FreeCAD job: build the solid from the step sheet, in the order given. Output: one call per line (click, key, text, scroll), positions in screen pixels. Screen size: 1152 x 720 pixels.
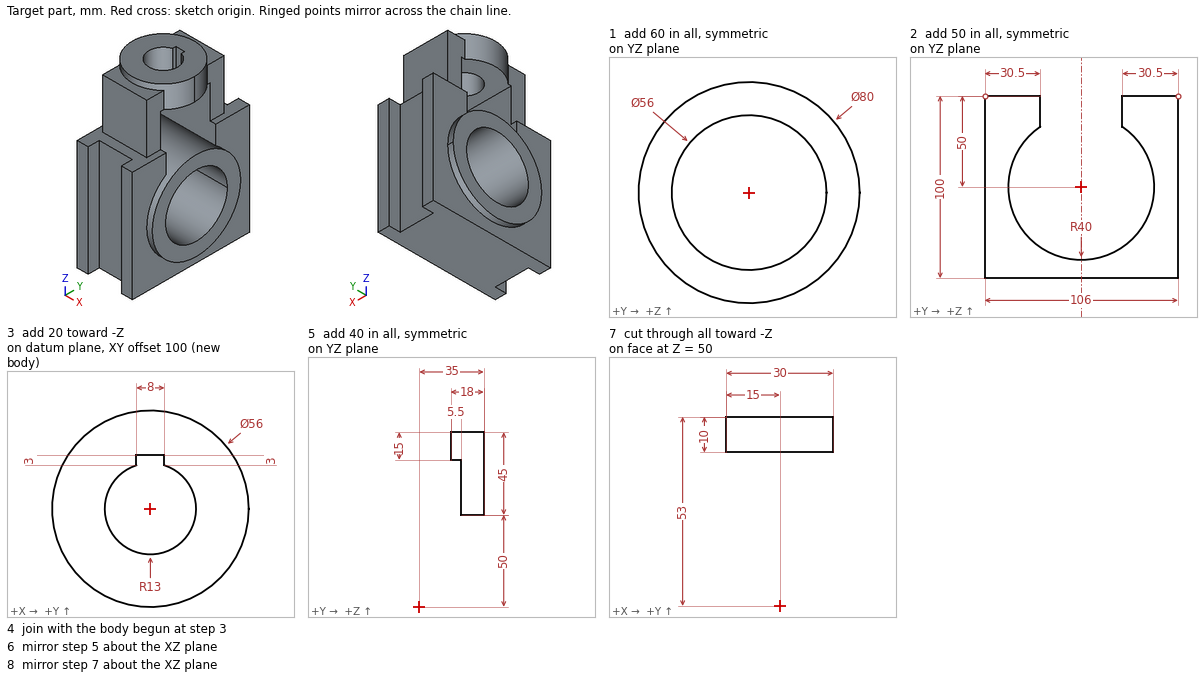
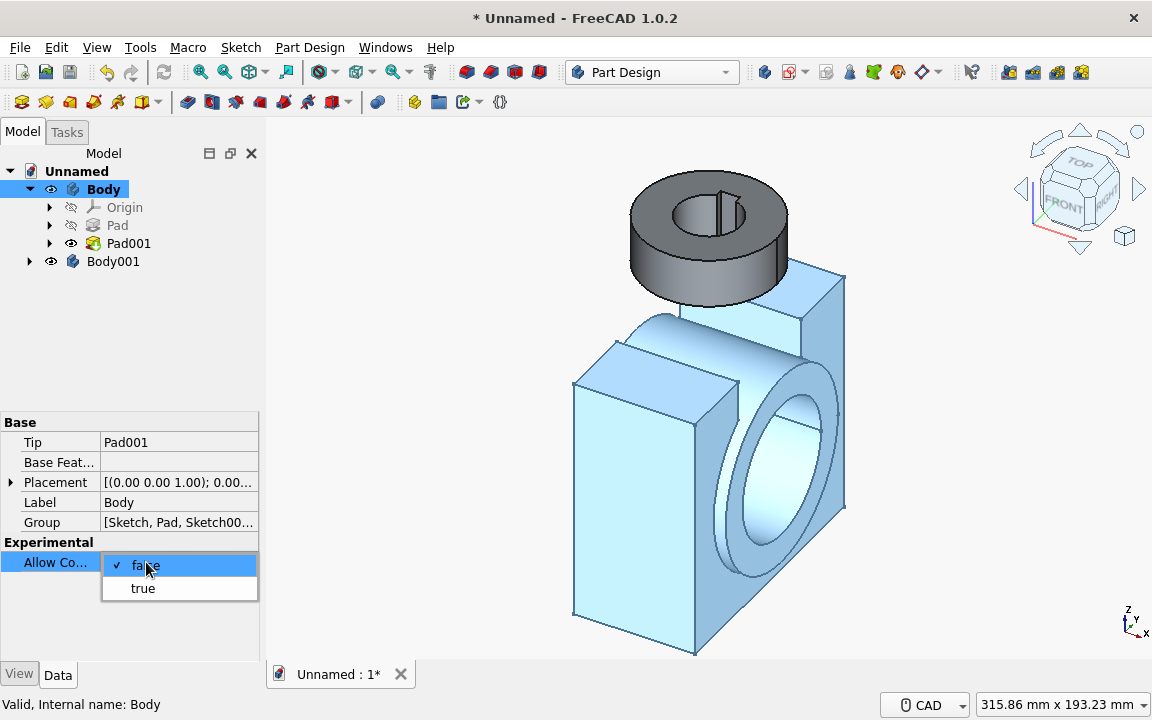
click(179, 588)
key(Return)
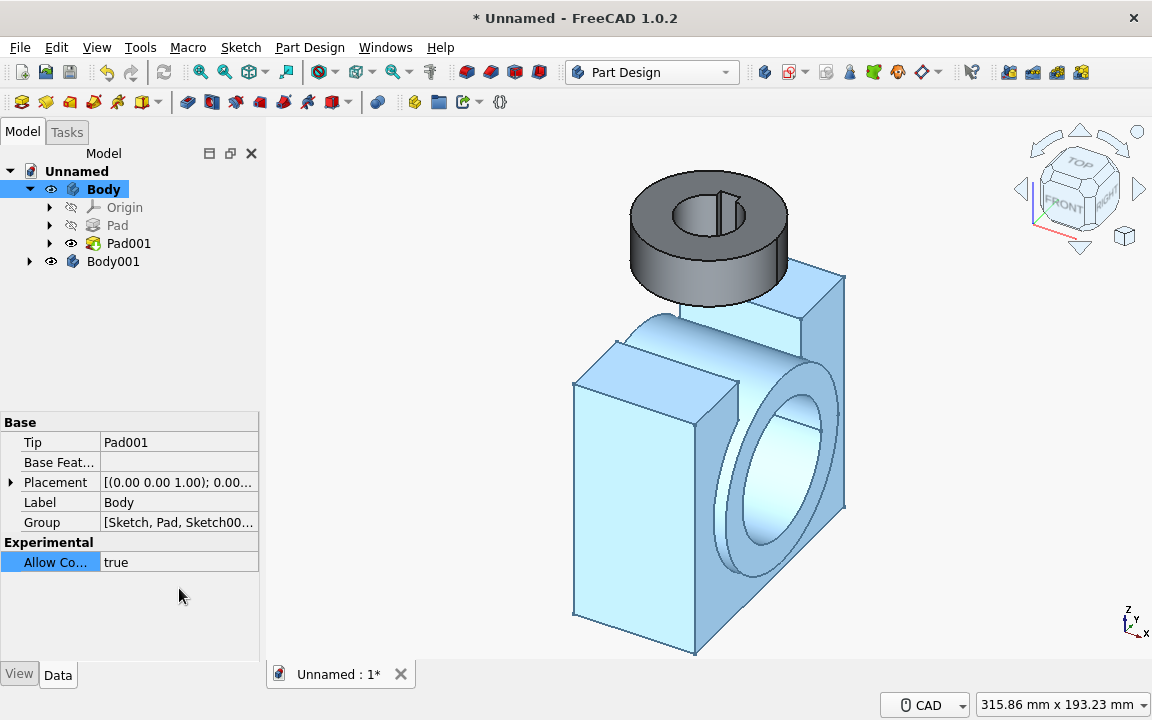
click(96, 261)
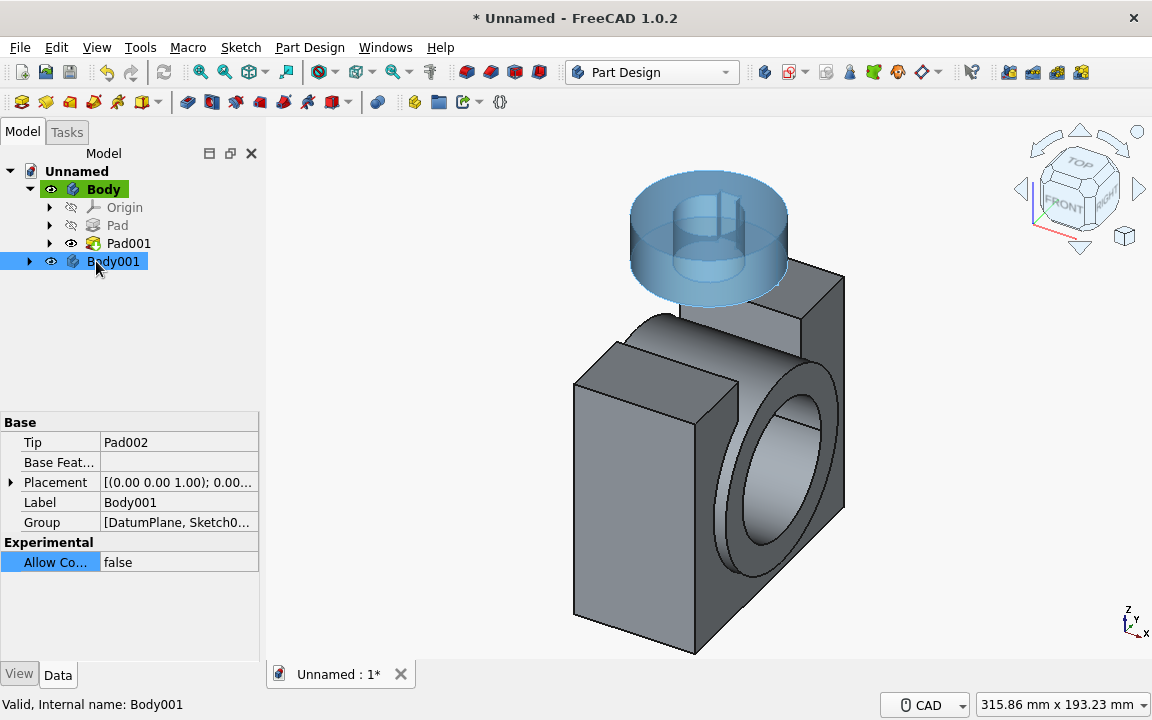
click(378, 102)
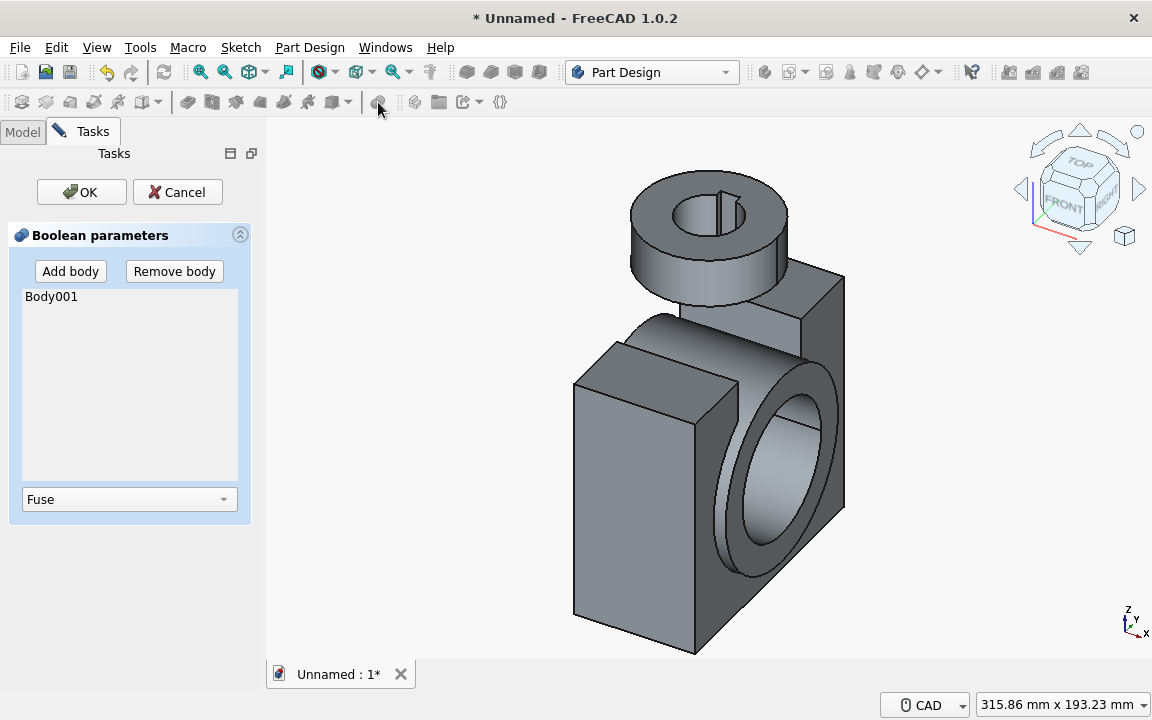
click(82, 192)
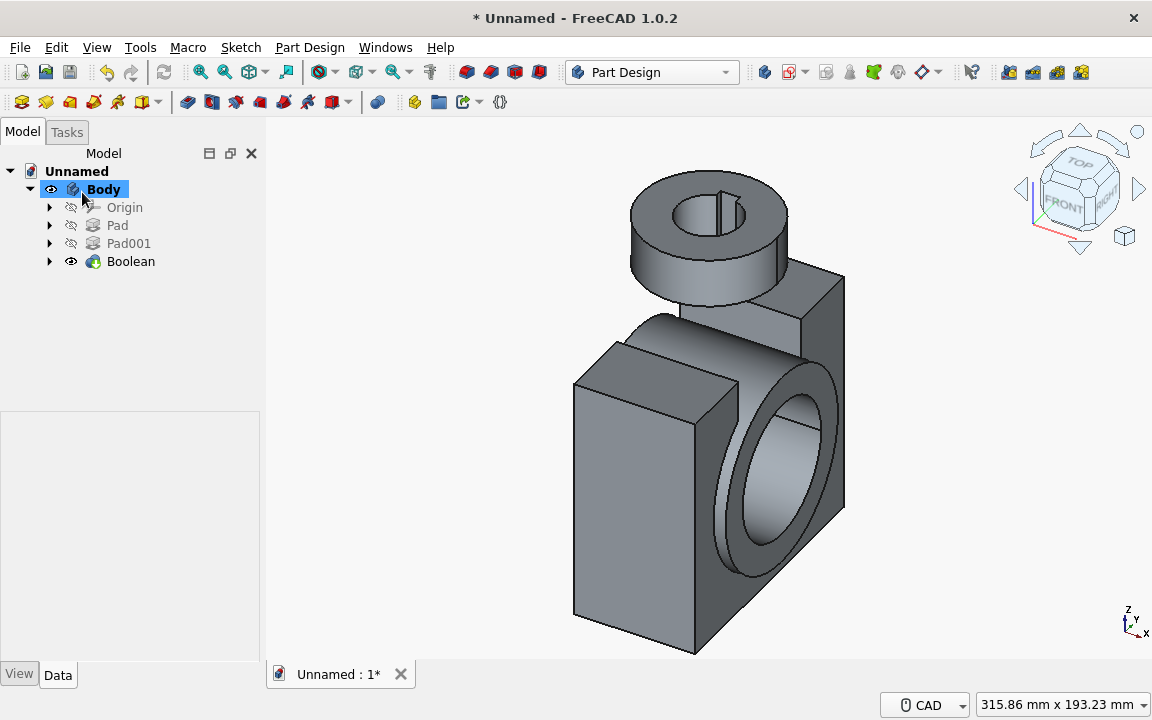
click(790, 72)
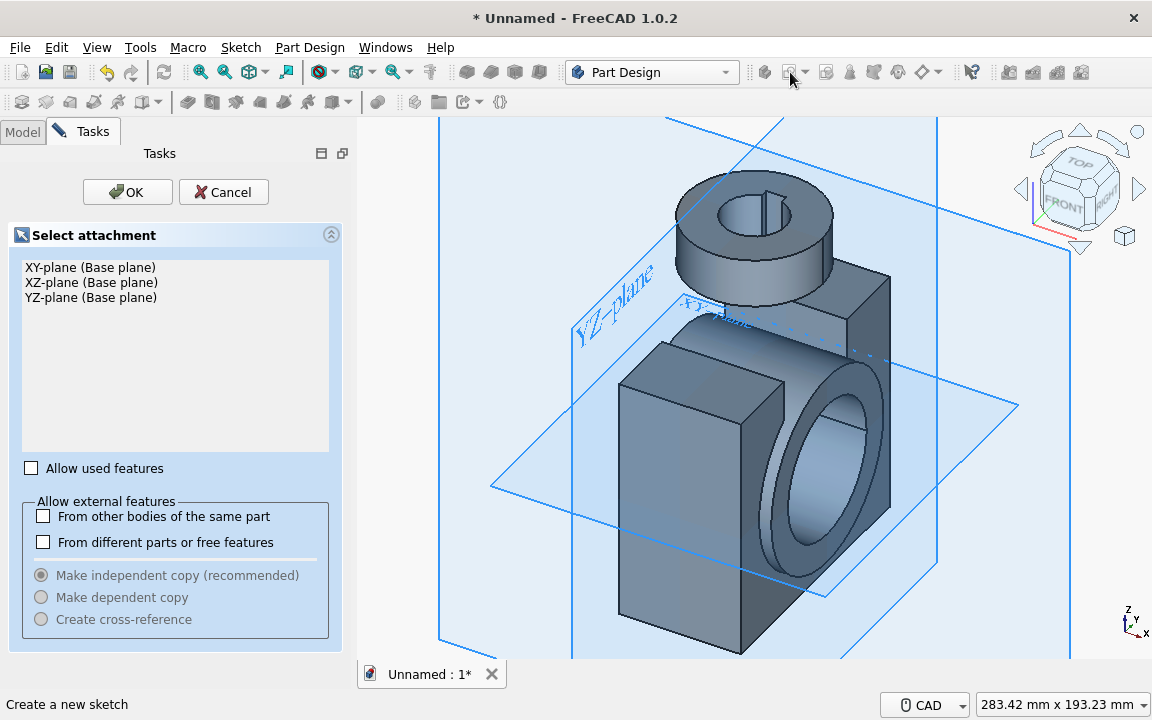
click(82, 298)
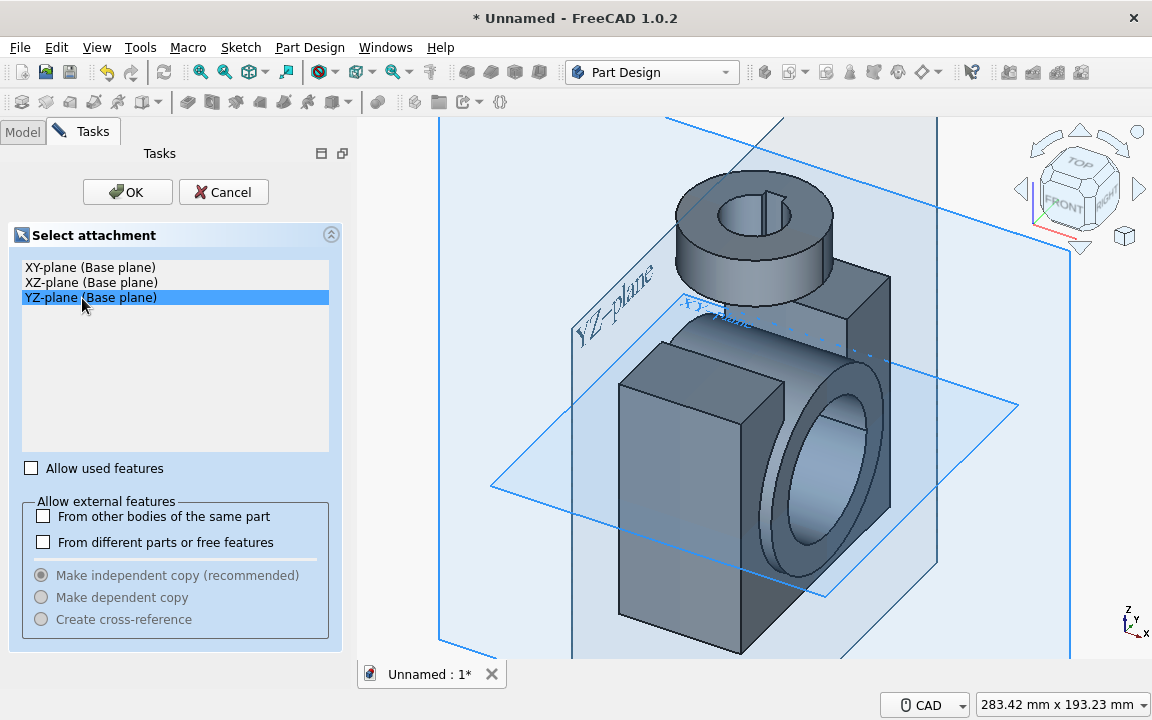
click(128, 192)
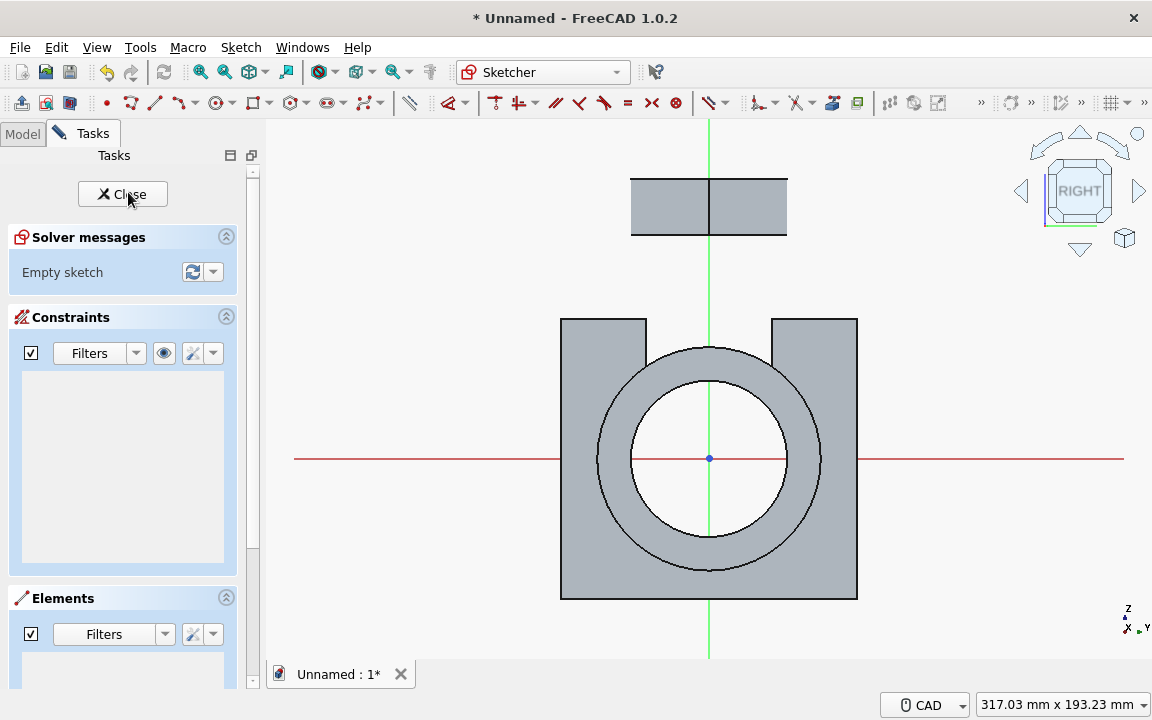
click(70, 104)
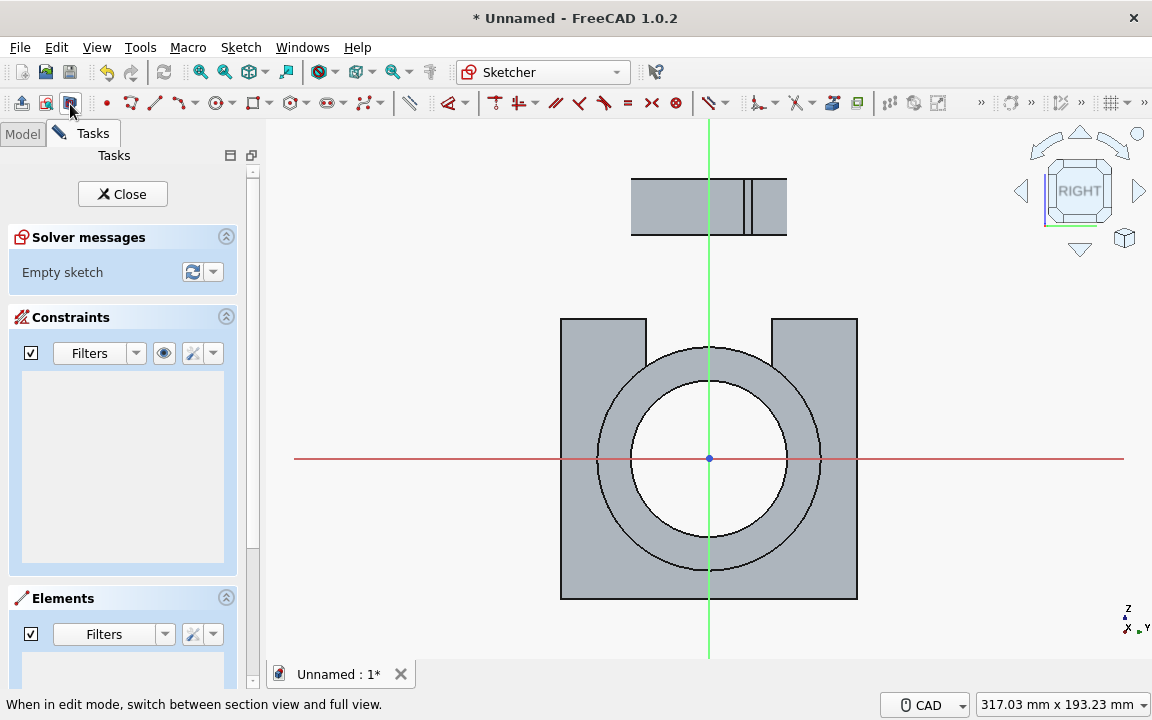
click(132, 104)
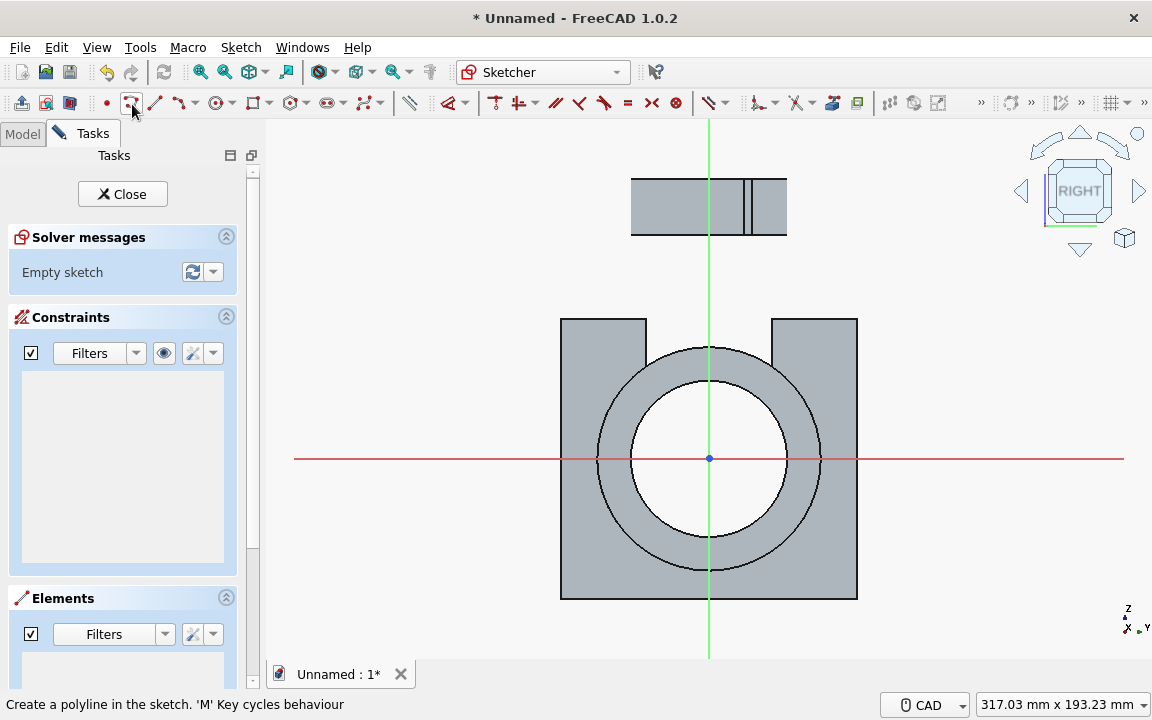
click(772, 319)
click(807, 319)
click(807, 193)
click(757, 193)
click(757, 235)
click(772, 235)
click(772, 320)
key(Escape)
key(Escape)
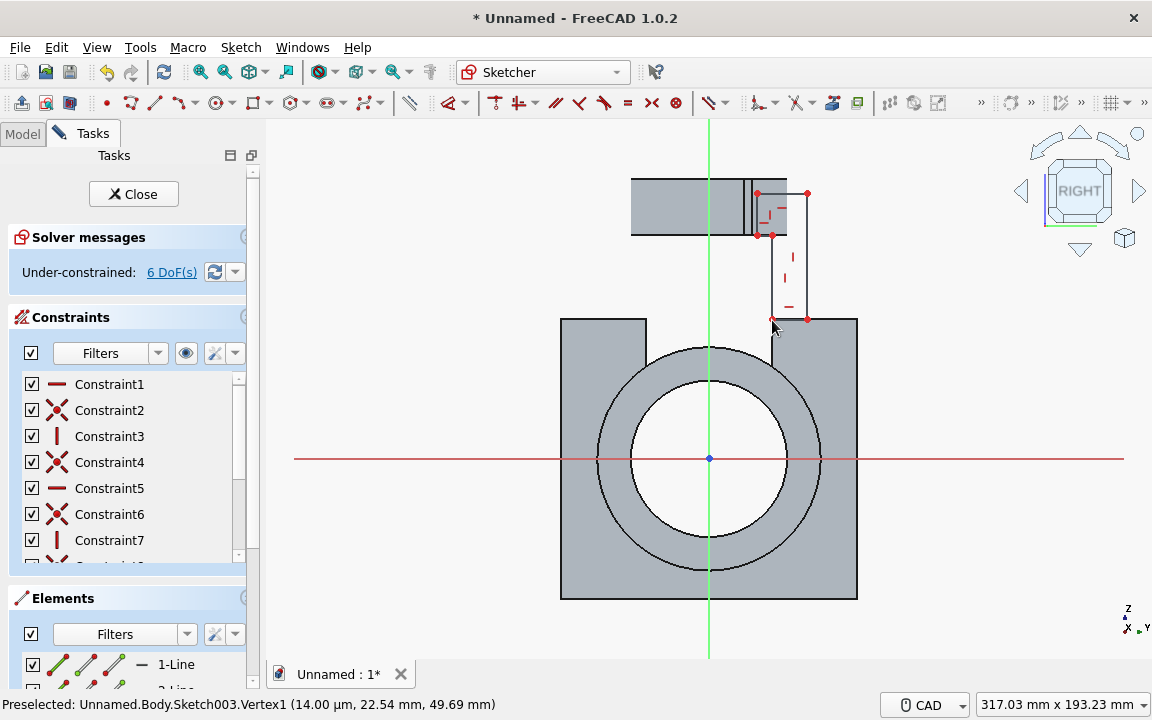
click(448, 104)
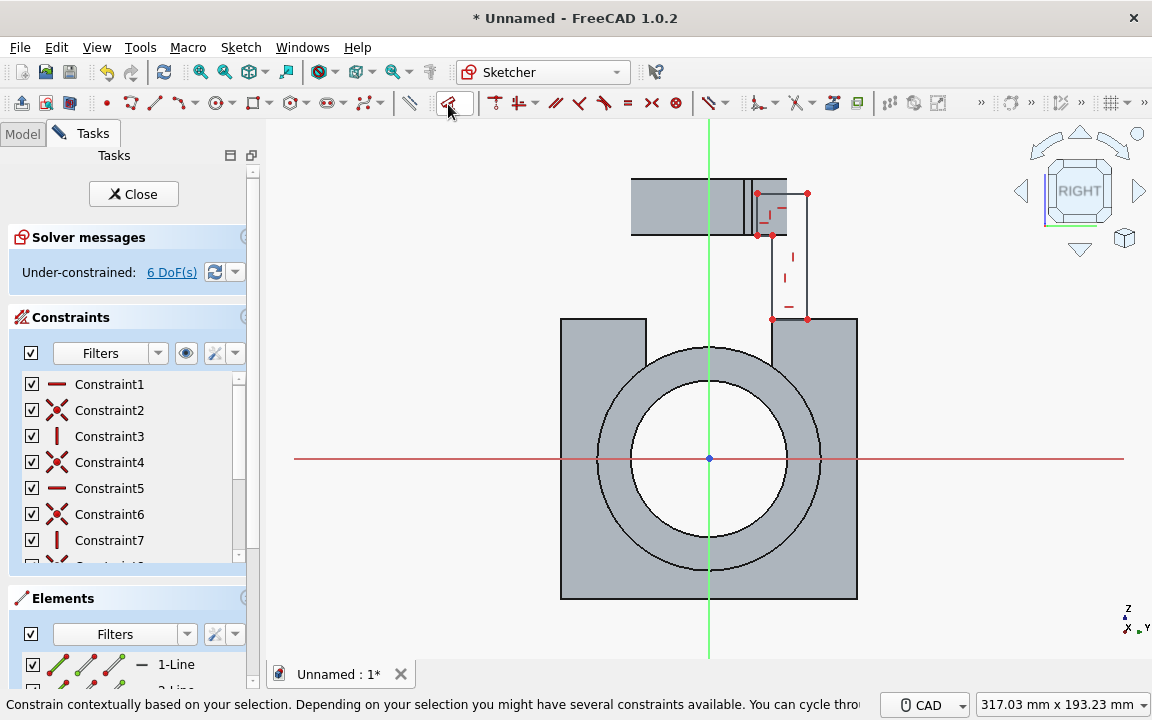
click(807, 282)
click(841, 257)